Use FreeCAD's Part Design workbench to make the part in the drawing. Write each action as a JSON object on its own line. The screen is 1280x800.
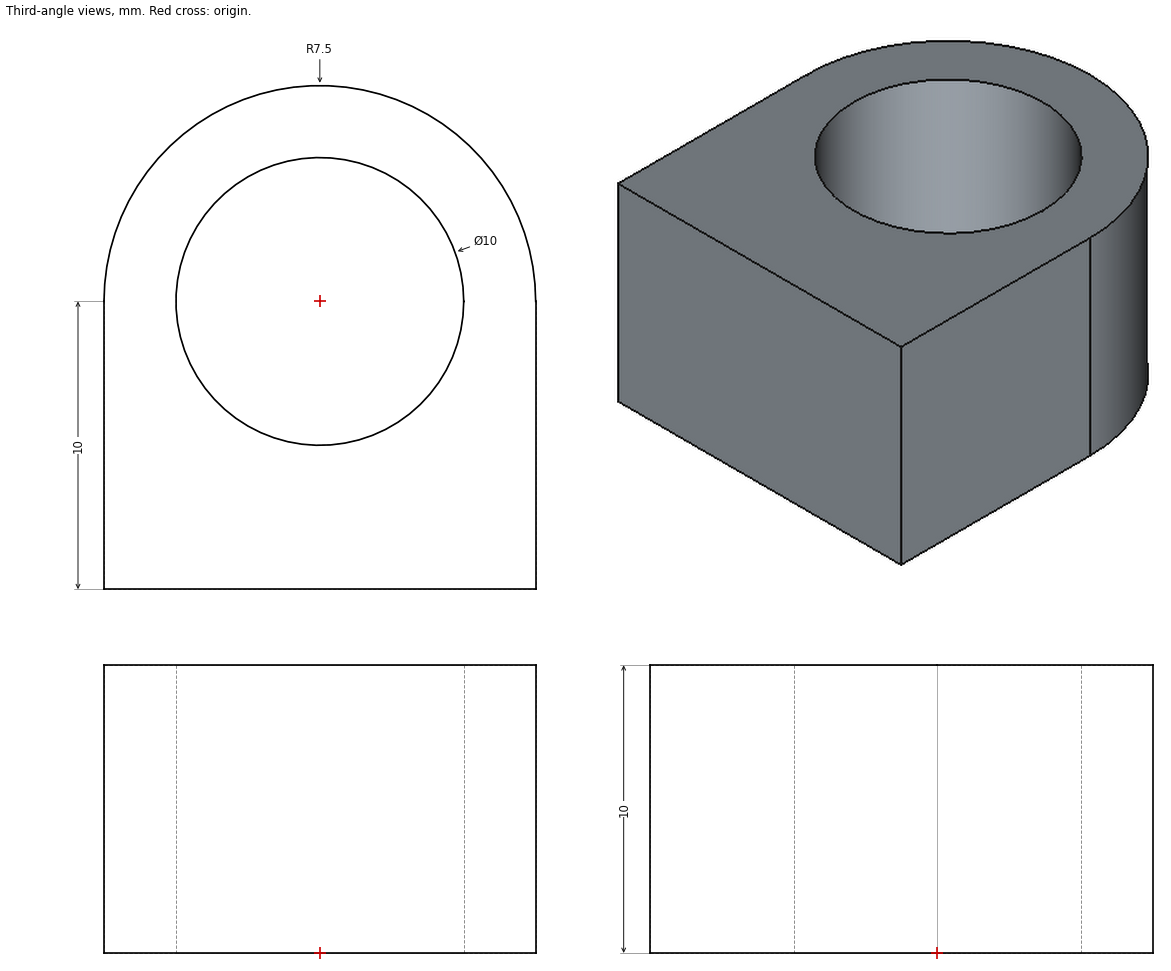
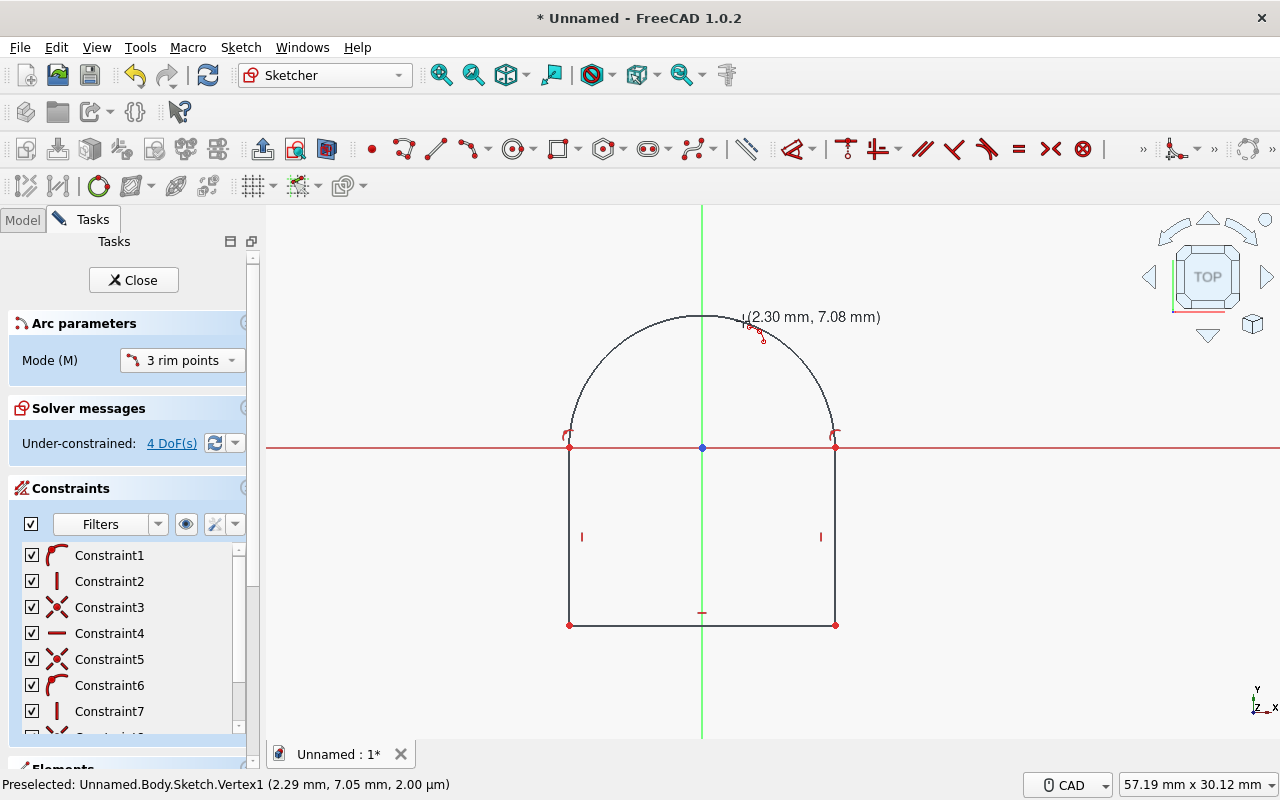
{"action": "left_click", "coordinate": [514, 150]}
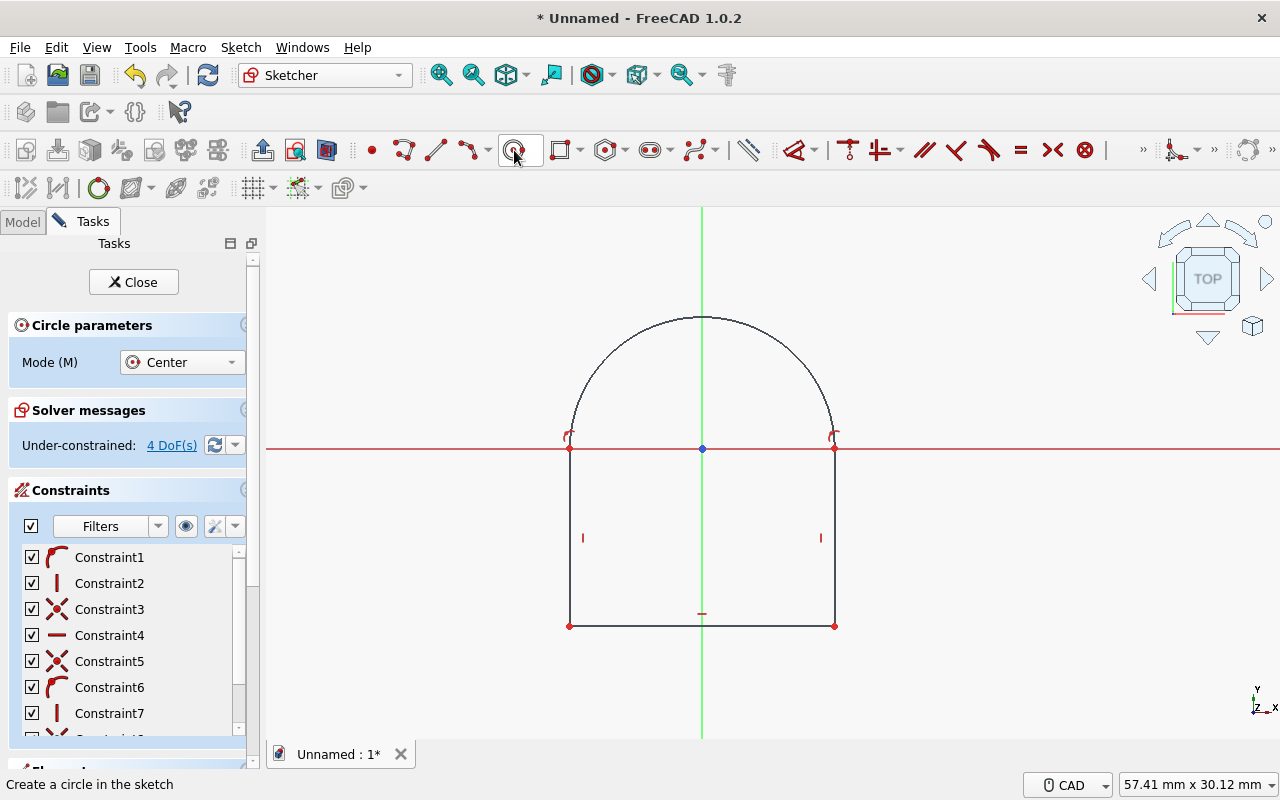
{"action": "left_click", "coordinate": [702, 449]}
{"action": "mouse_move", "coordinate": [765, 386]}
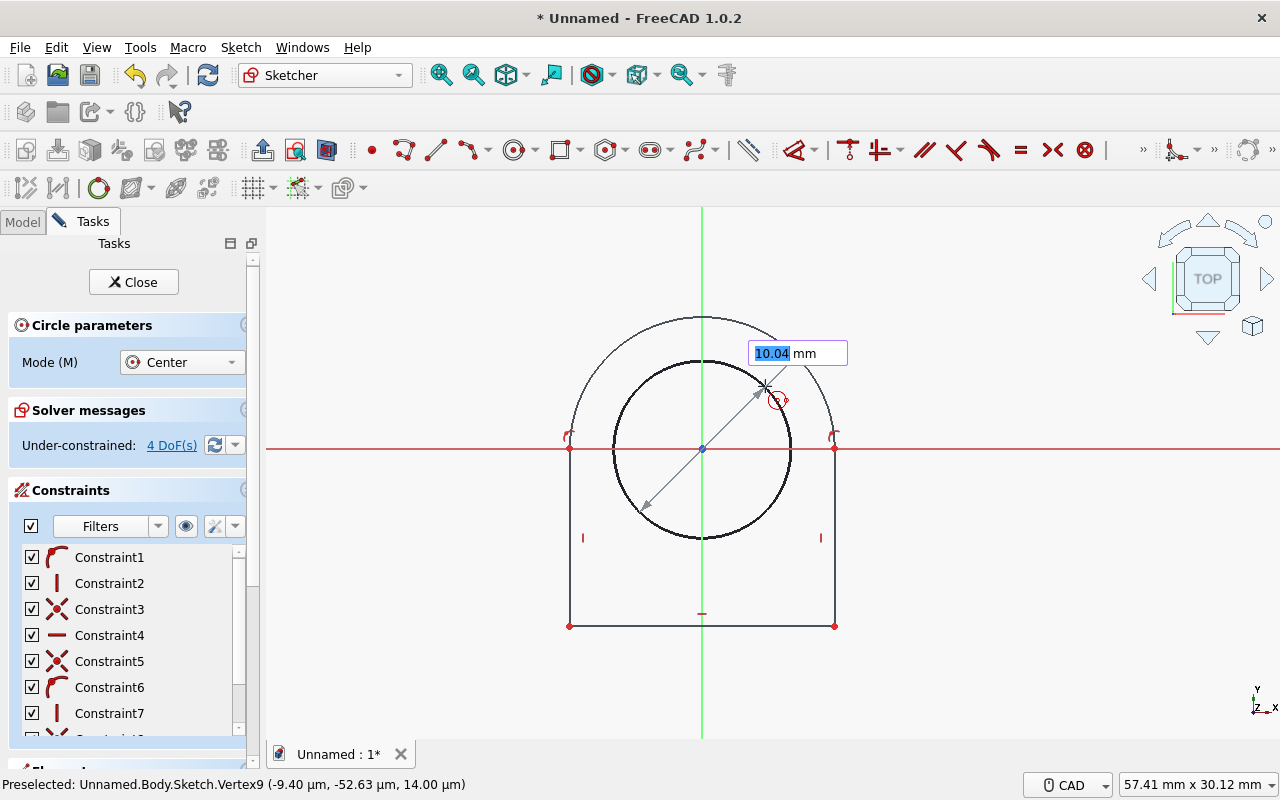
{"action": "type", "text": "10"}
{"action": "key", "text": "Return"}
{"action": "key", "text": "Escape"}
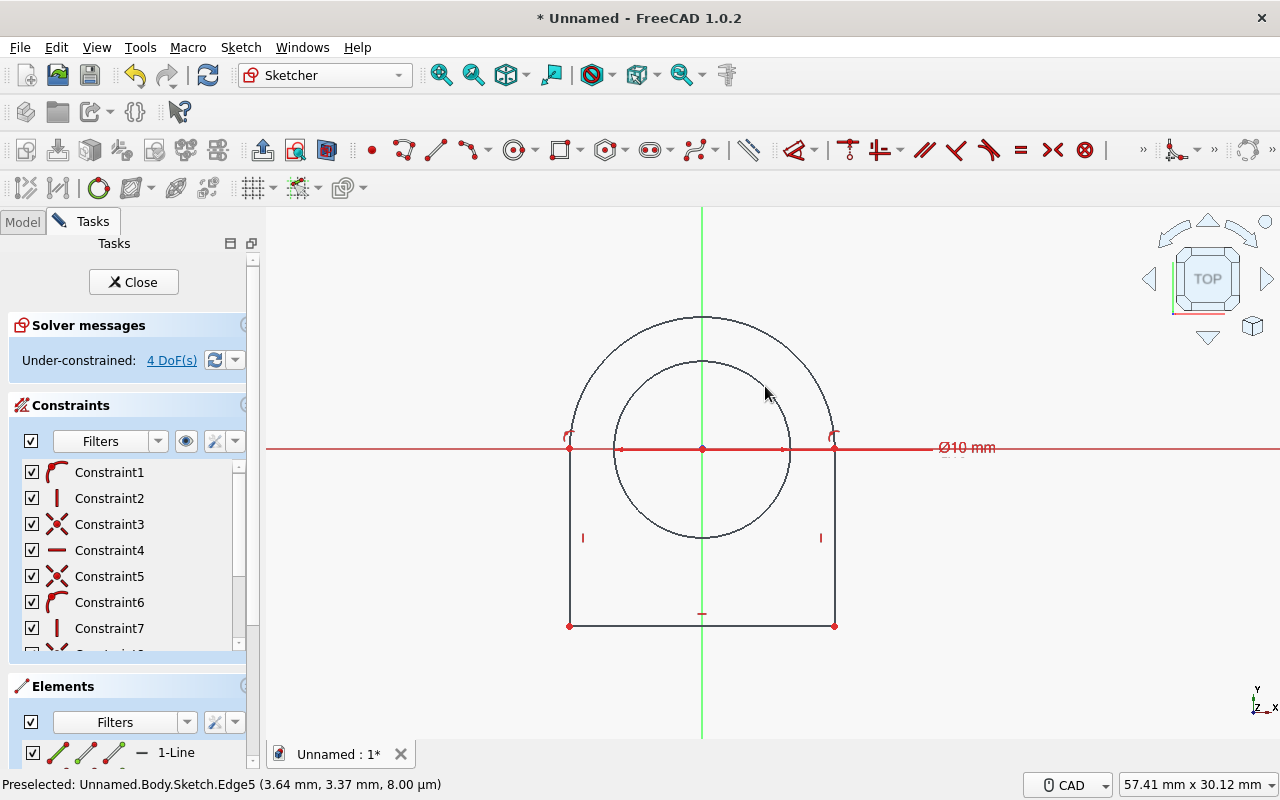
{"action": "left_click", "coordinate": [570, 502]}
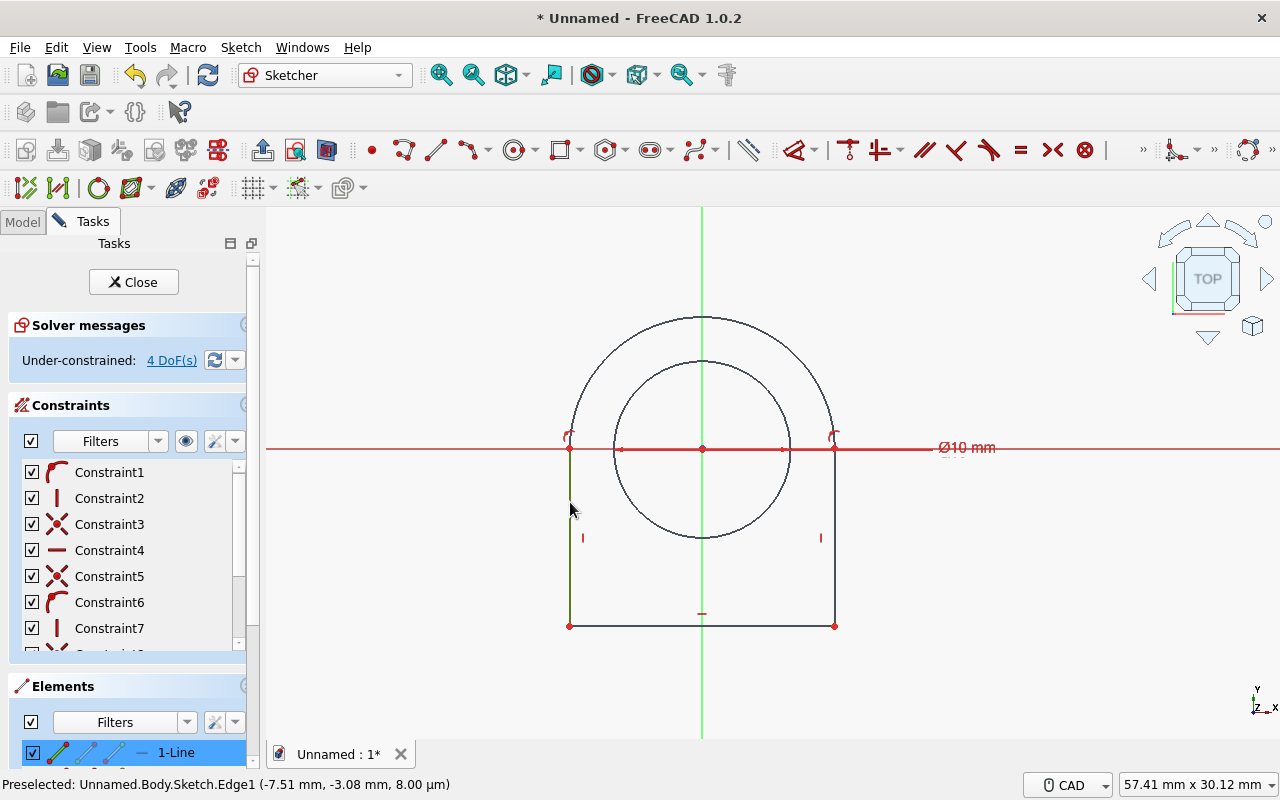
{"action": "left_click", "coordinate": [780, 342]}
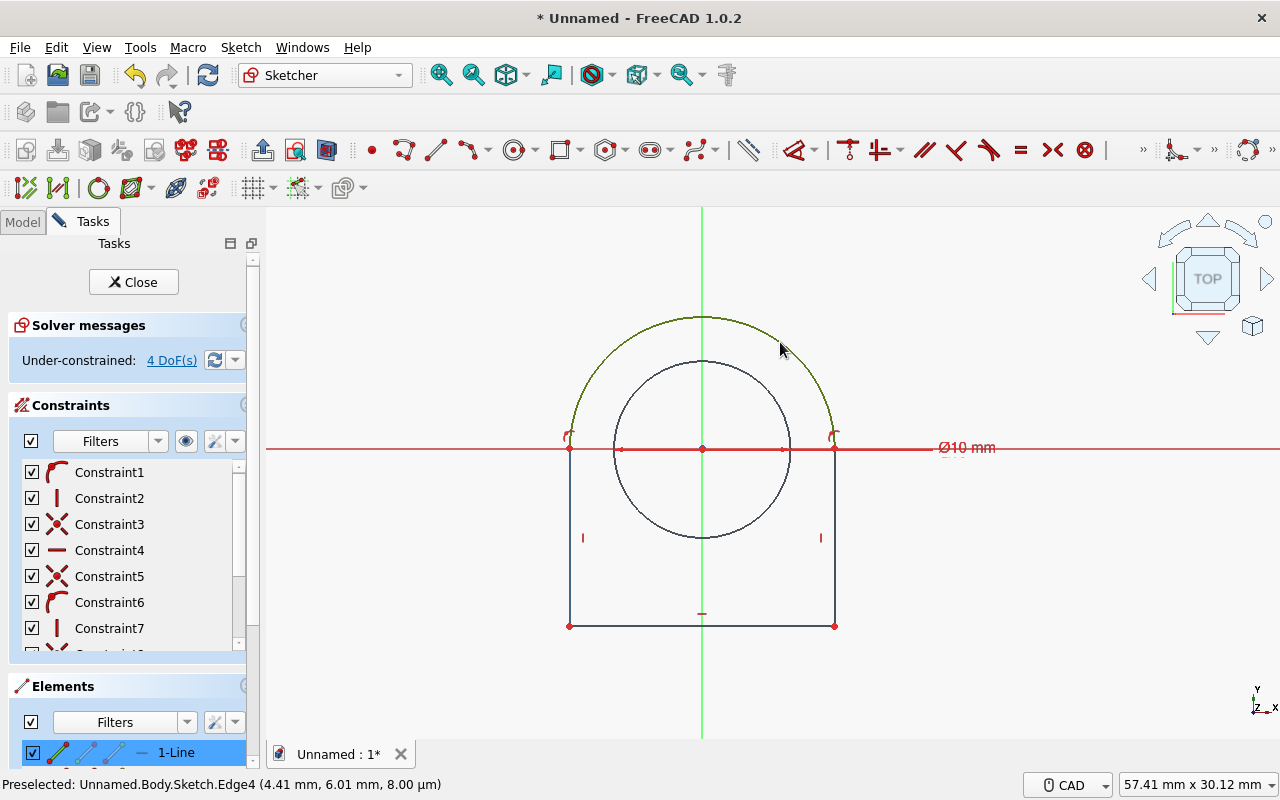
{"action": "left_click", "coordinate": [990, 150]}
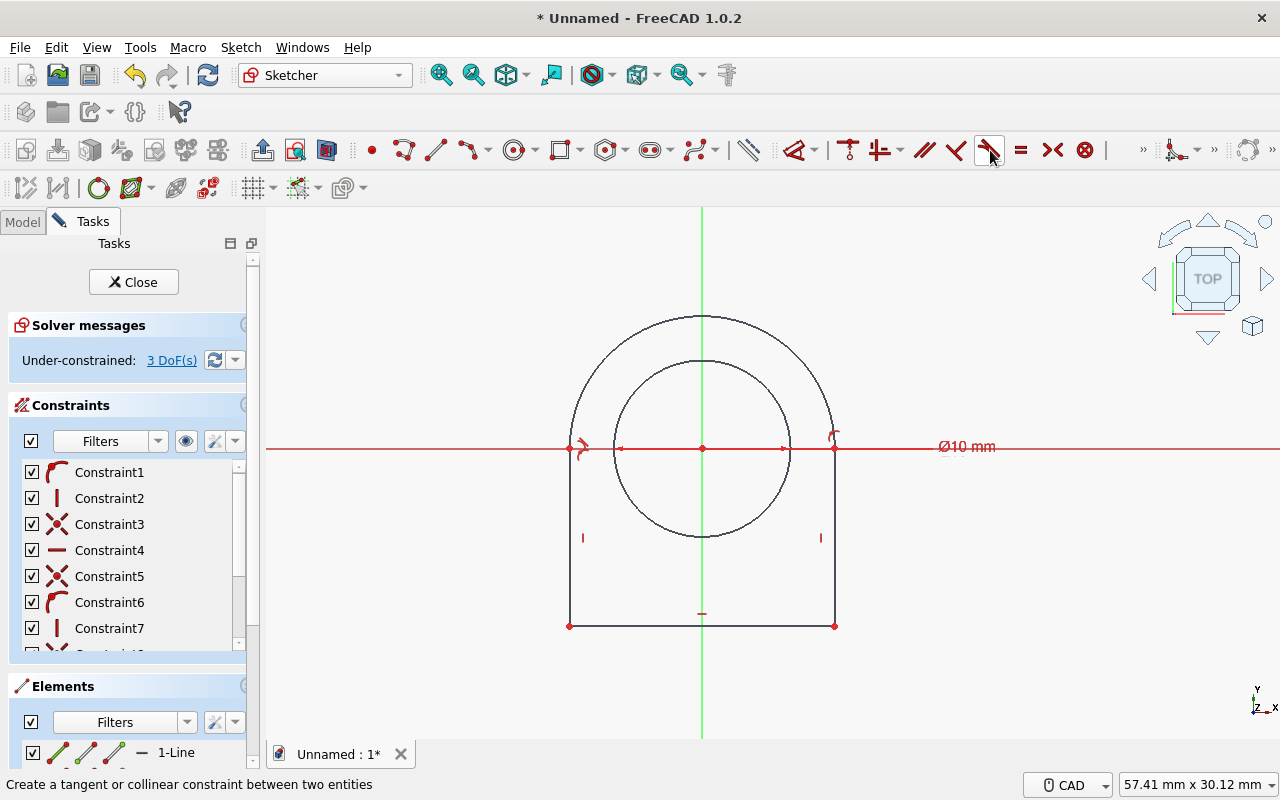
{"action": "left_click", "coordinate": [702, 449]}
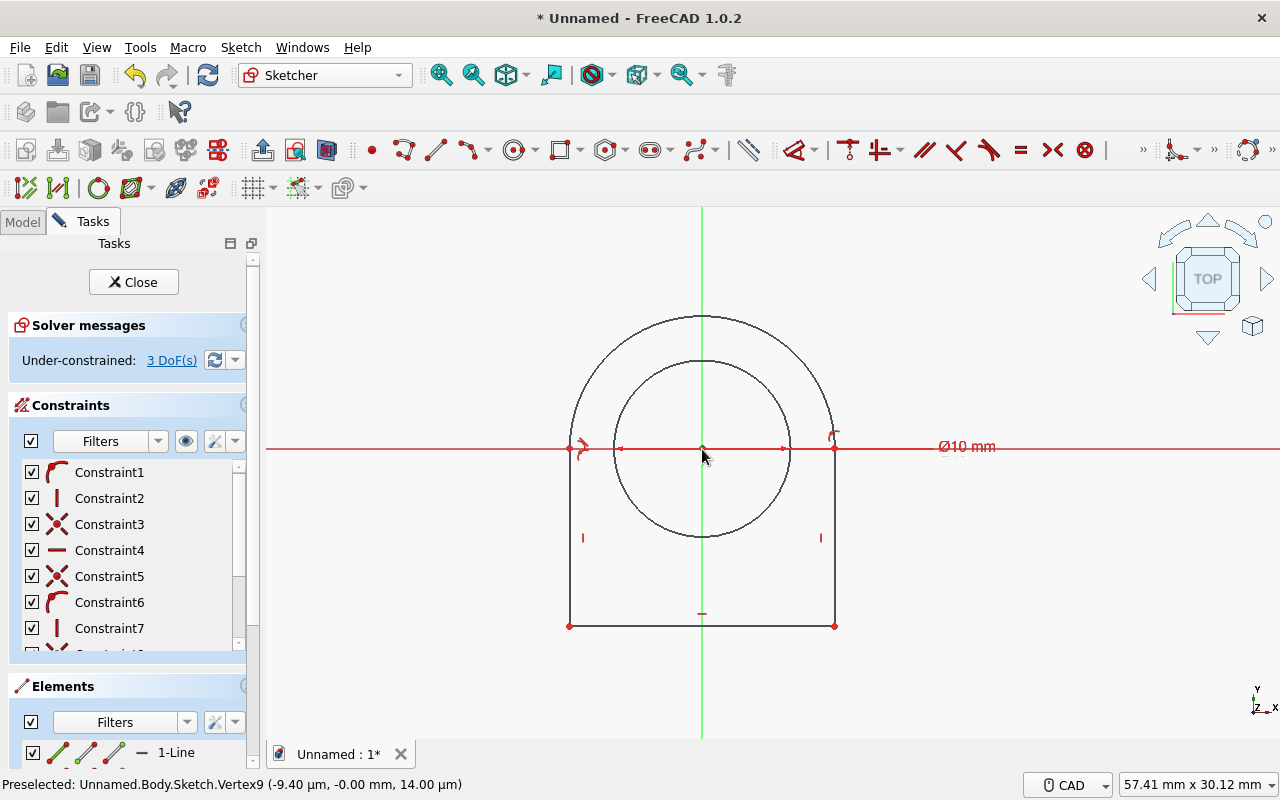
{"action": "left_click", "coordinate": [702, 677]}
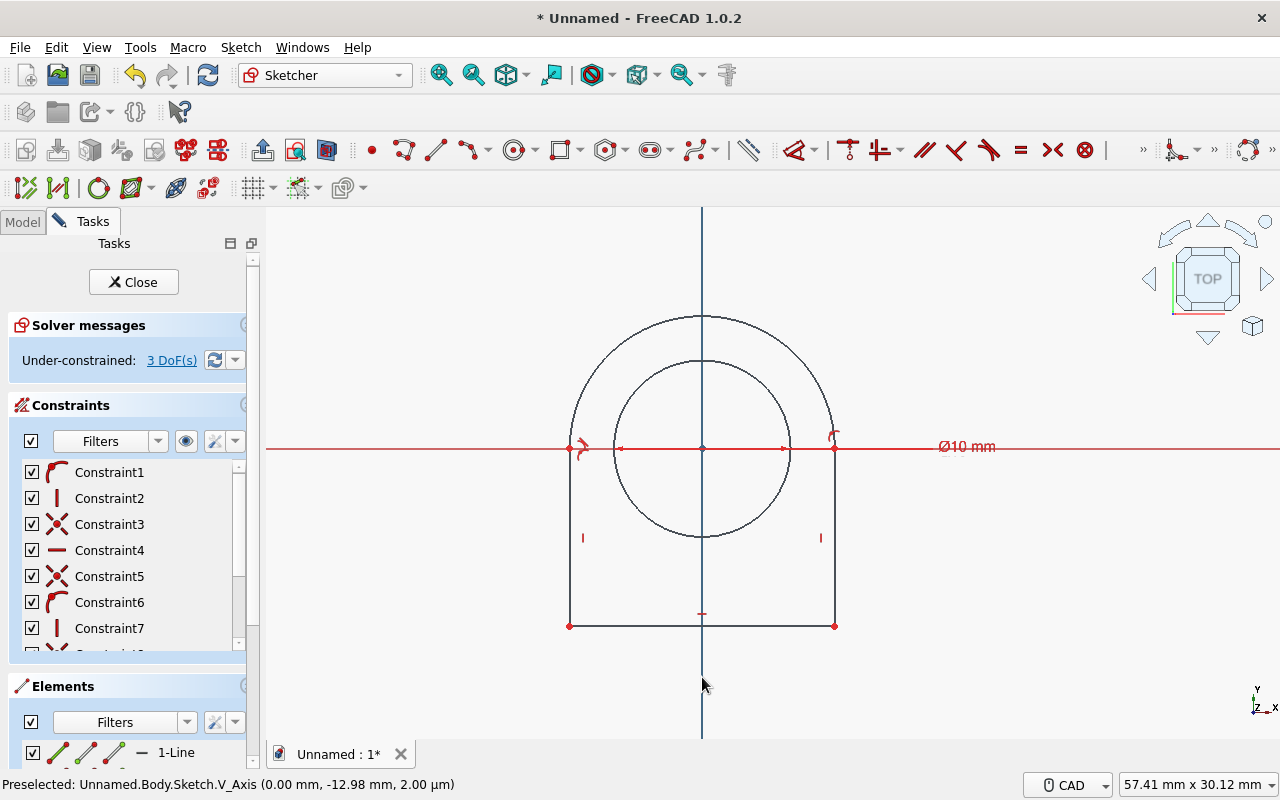
{"action": "left_click", "coordinate": [848, 150]}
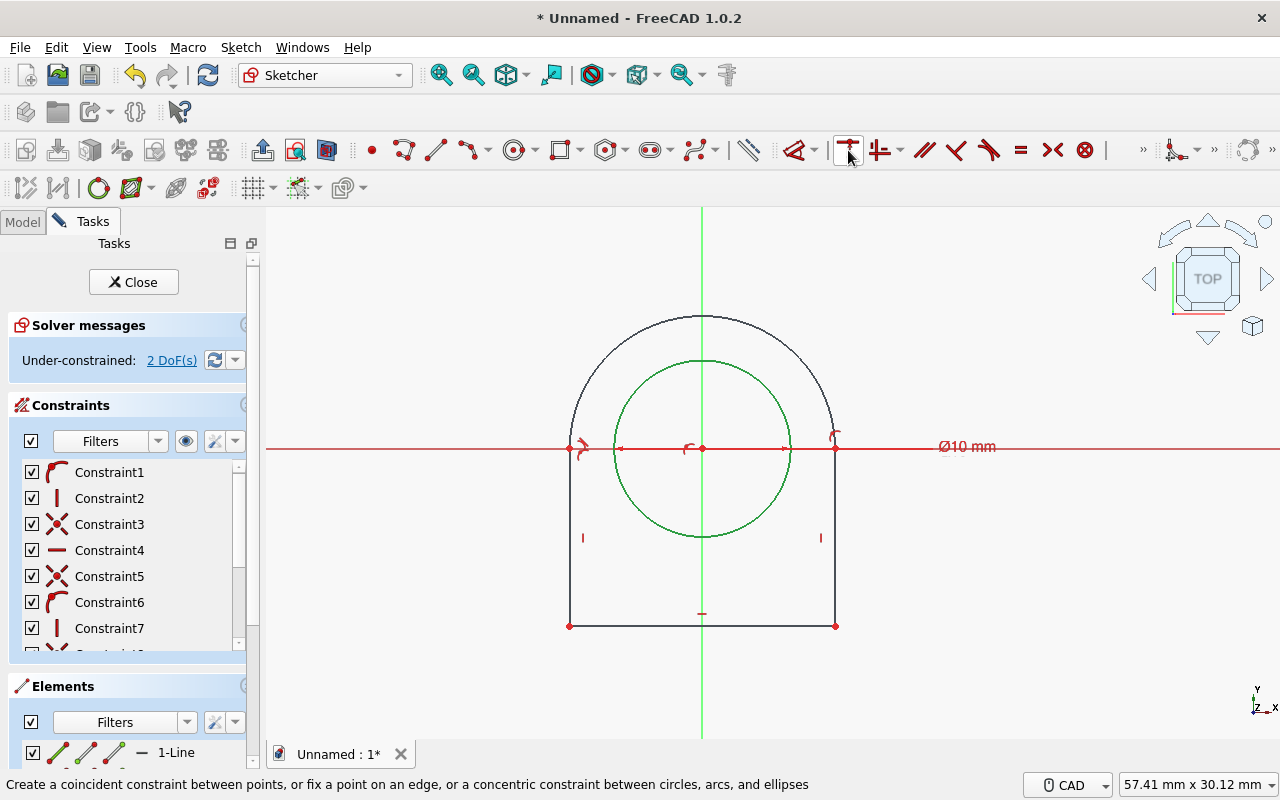
{"action": "left_click", "coordinate": [780, 341]}